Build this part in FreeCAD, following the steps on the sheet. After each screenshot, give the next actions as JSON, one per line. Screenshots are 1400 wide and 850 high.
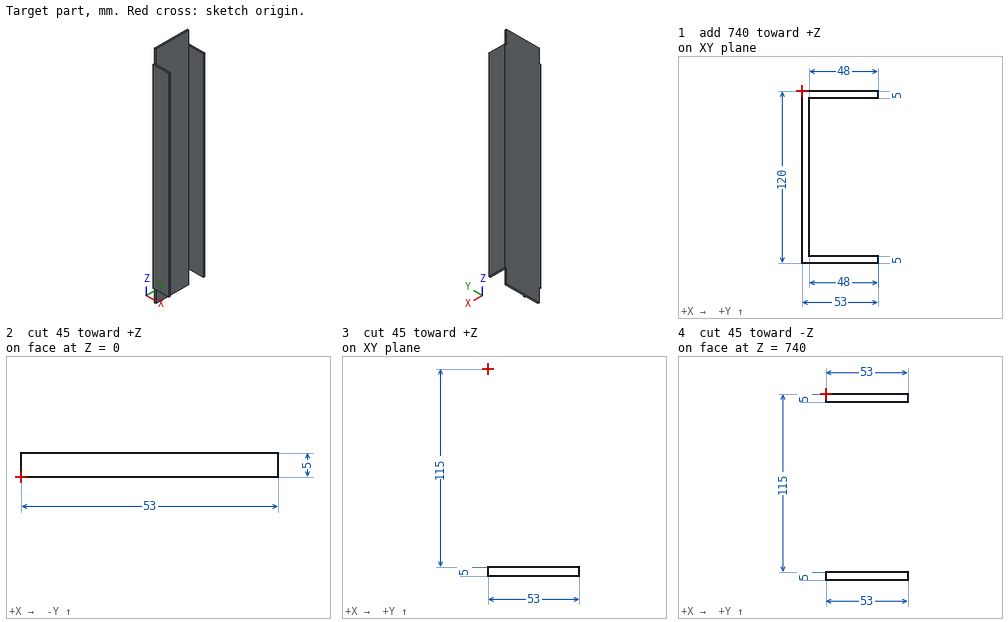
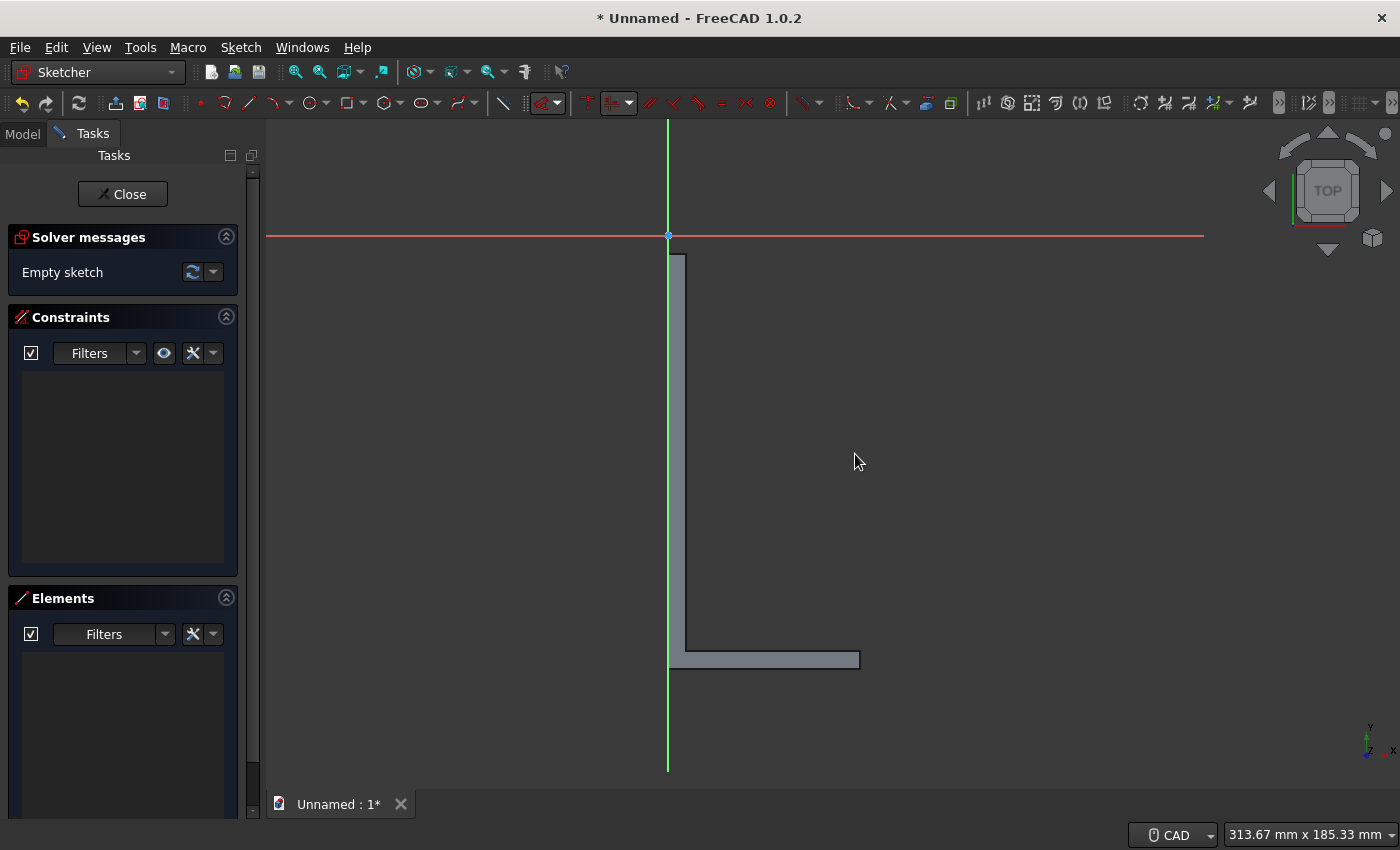
{"action": "left_click", "coordinate": [348, 104]}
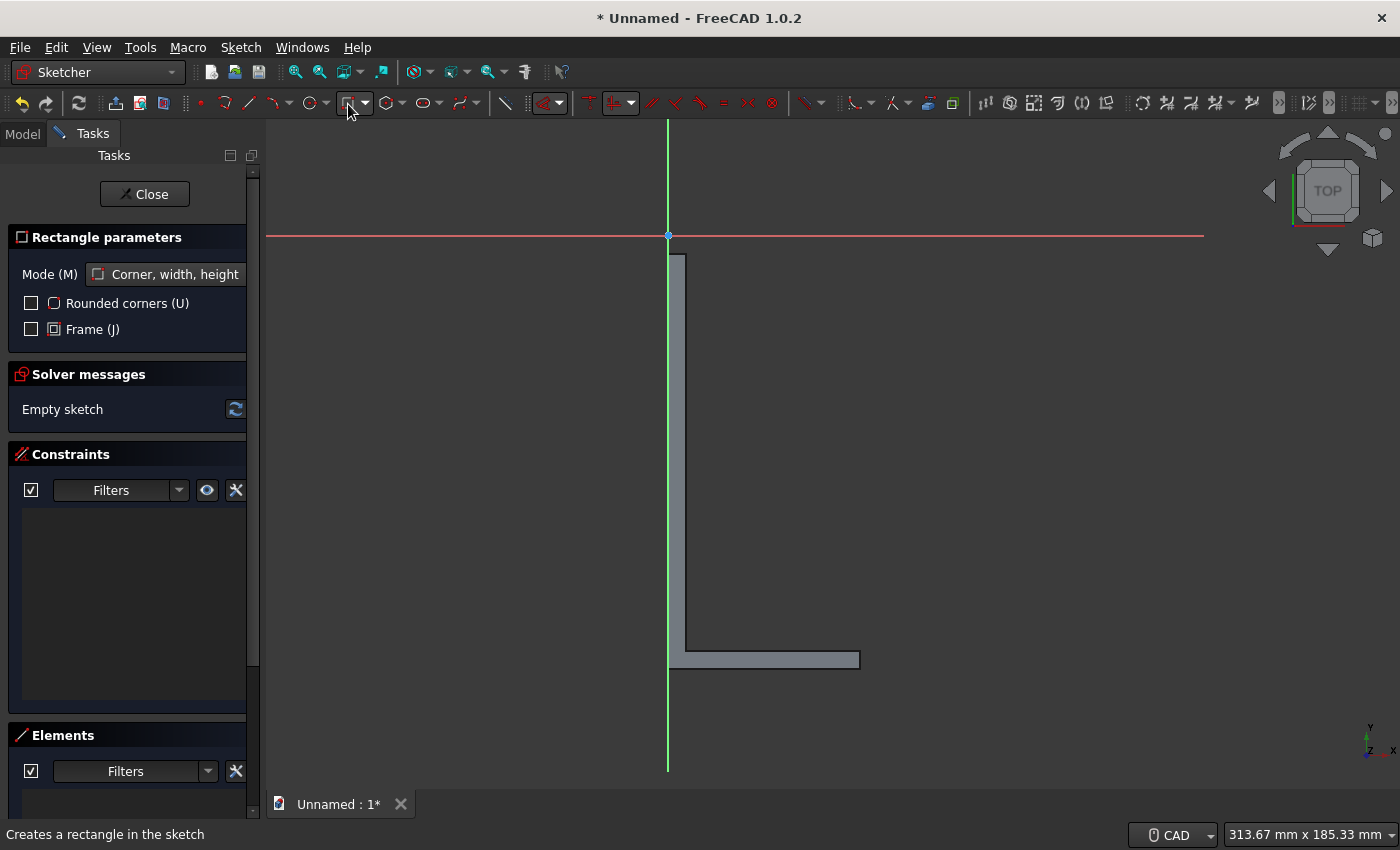
{"action": "left_click", "coordinate": [668, 651]}
{"action": "left_click", "coordinate": [860, 669]}
{"action": "key", "text": "Escape"}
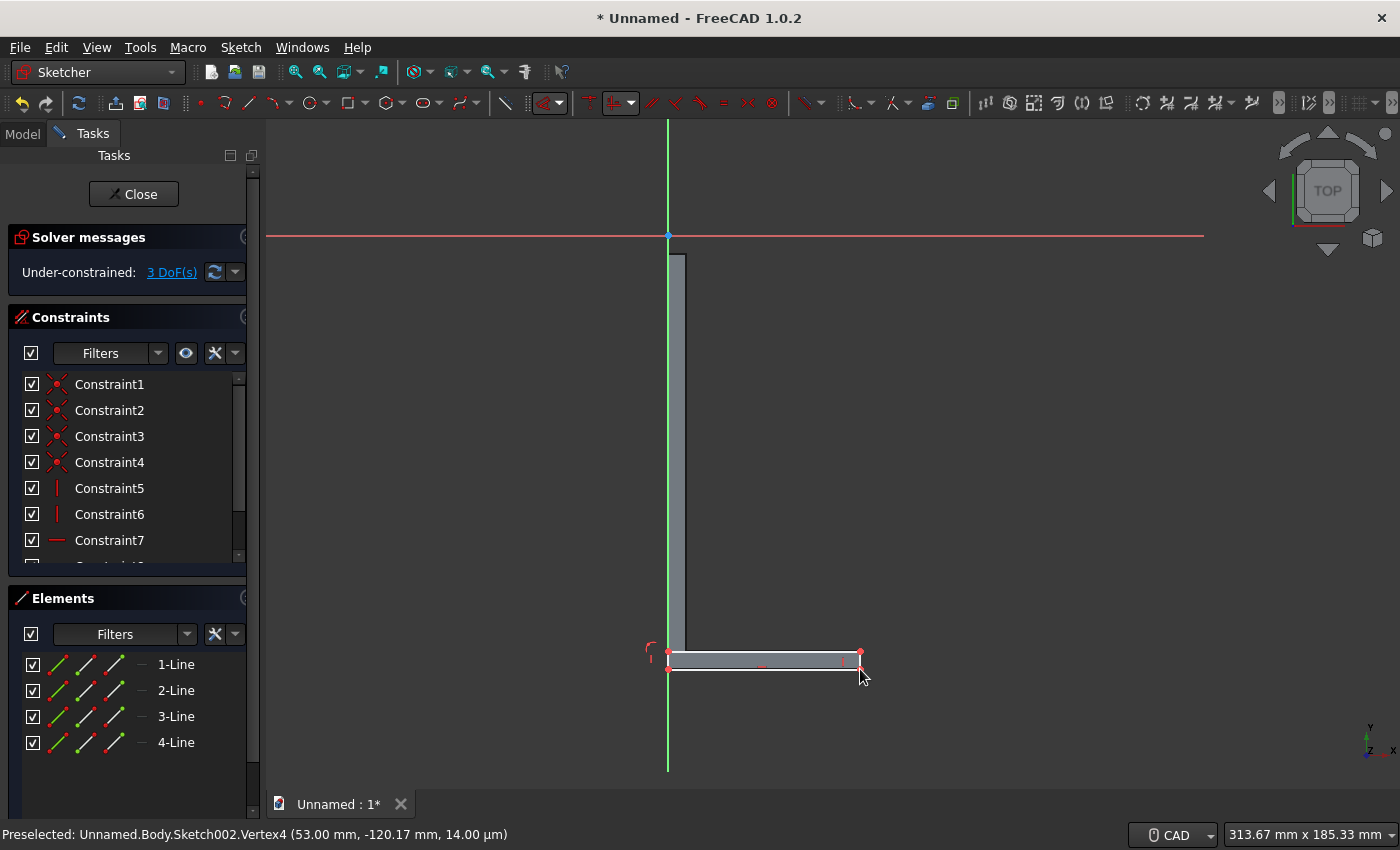
{"action": "scroll", "coordinate": [668, 661], "scroll_direction": "up", "scroll_amount": 4}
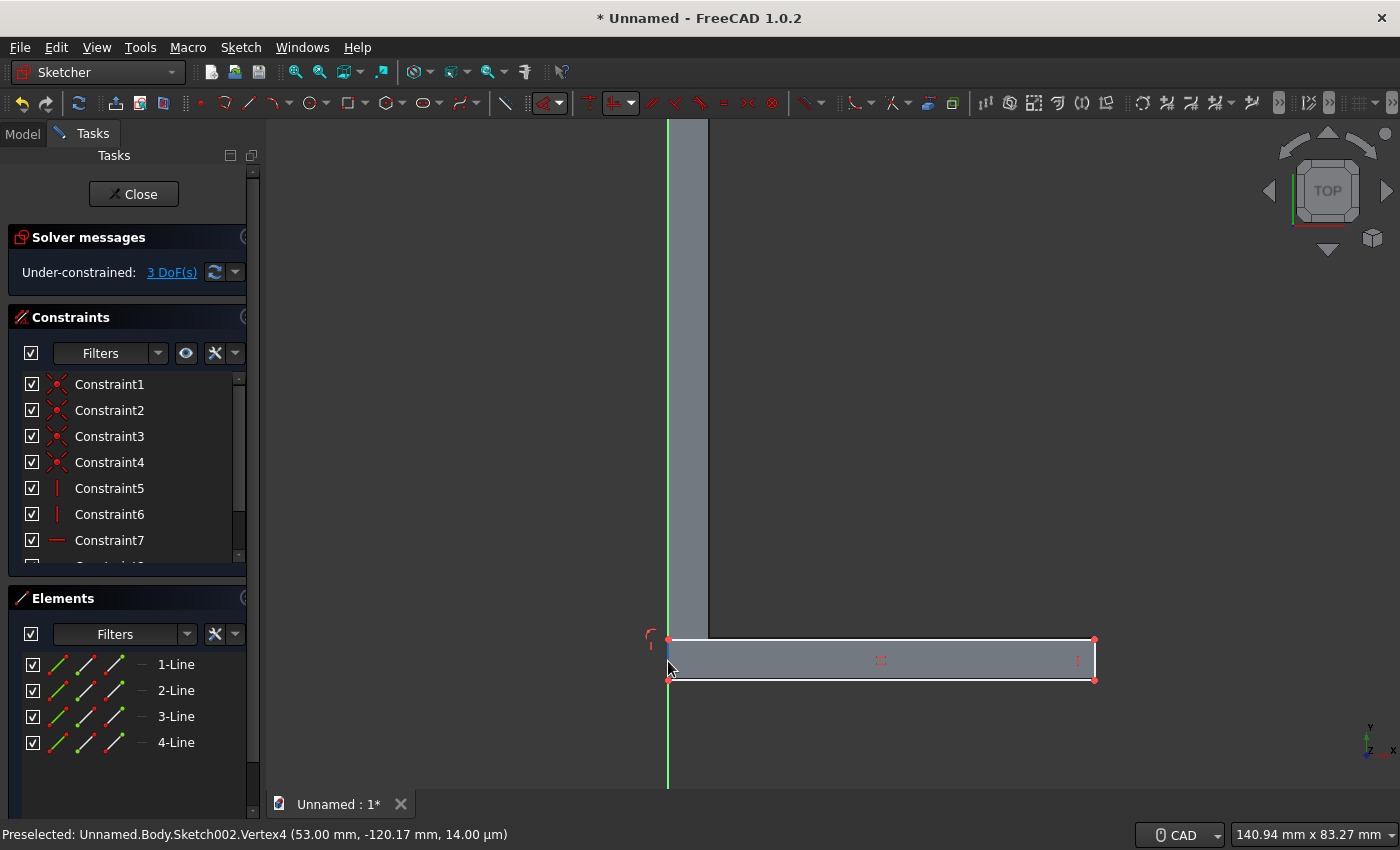
{"action": "left_click", "coordinate": [668, 660]}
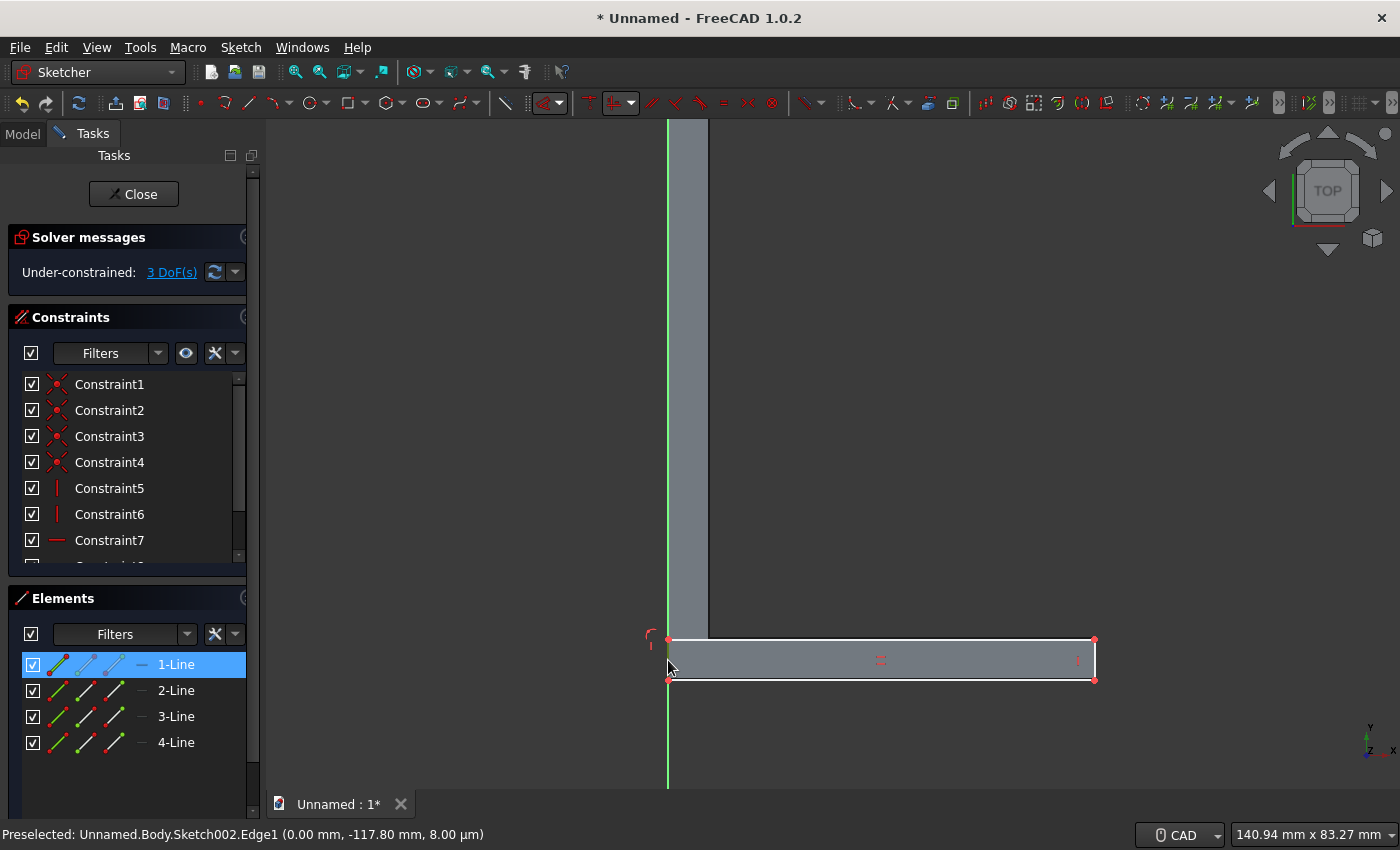
{"action": "left_click", "coordinate": [562, 104]}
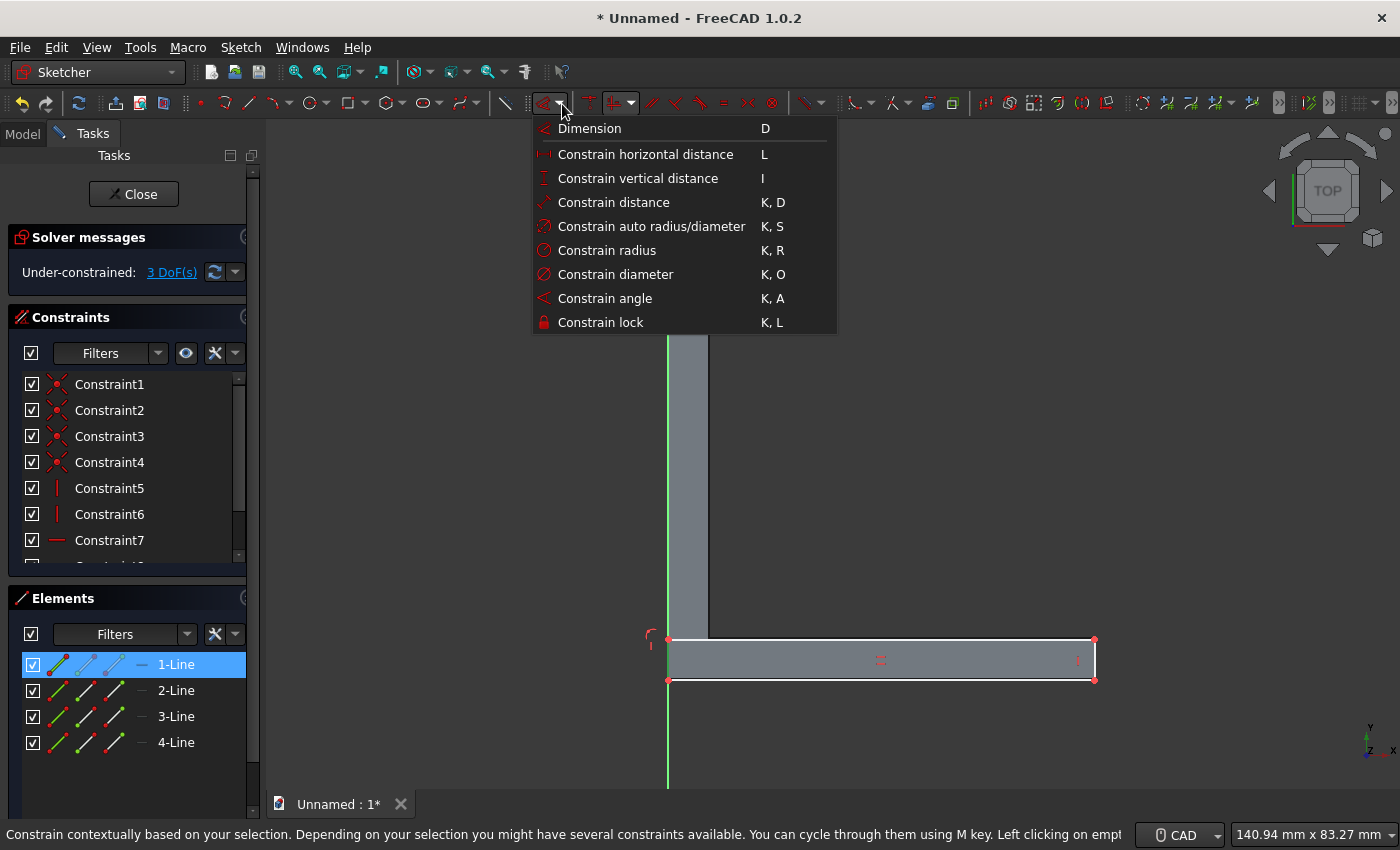
{"action": "left_click", "coordinate": [685, 178]}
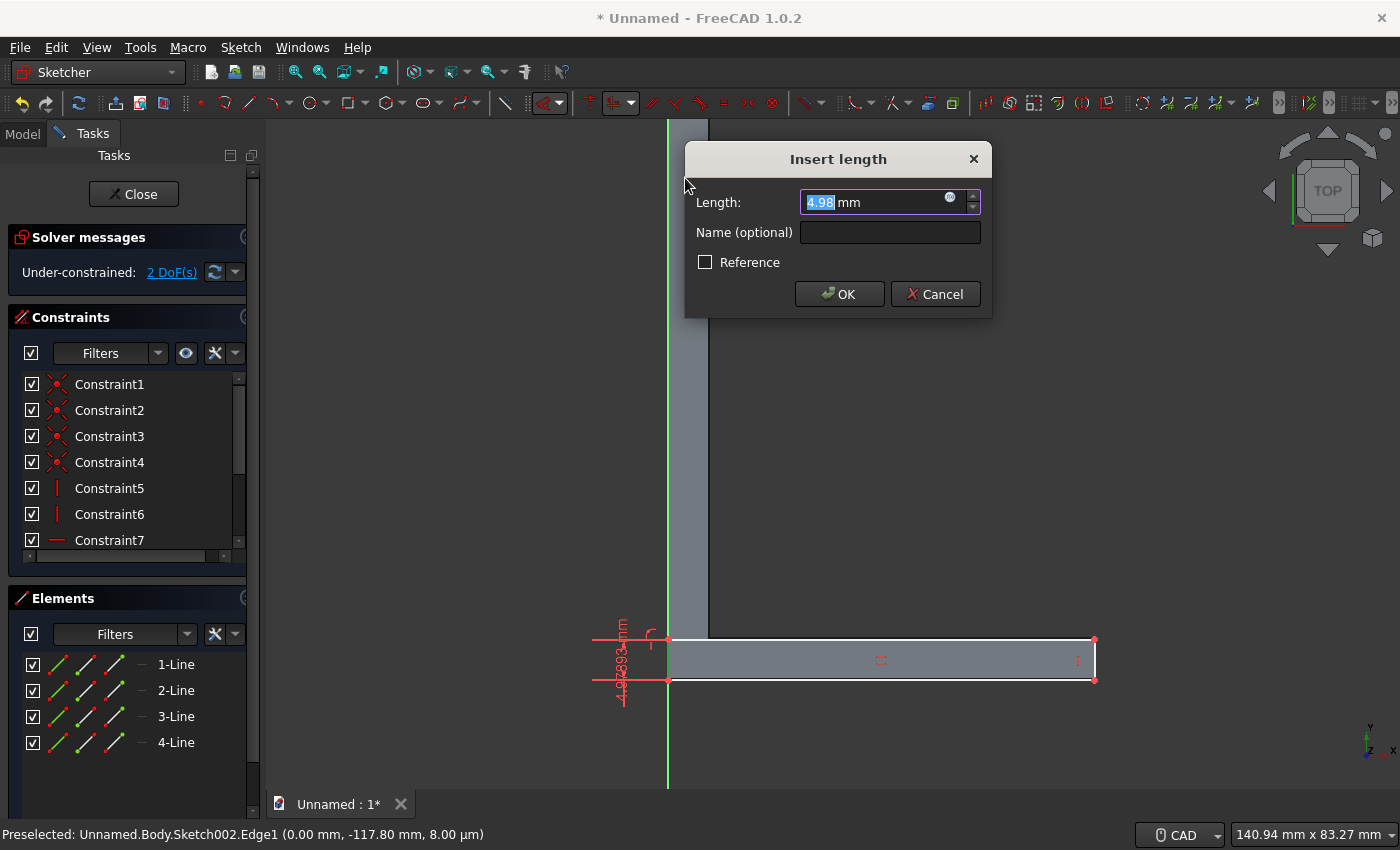
{"action": "type", "text": "5"}
{"action": "key", "text": "Return"}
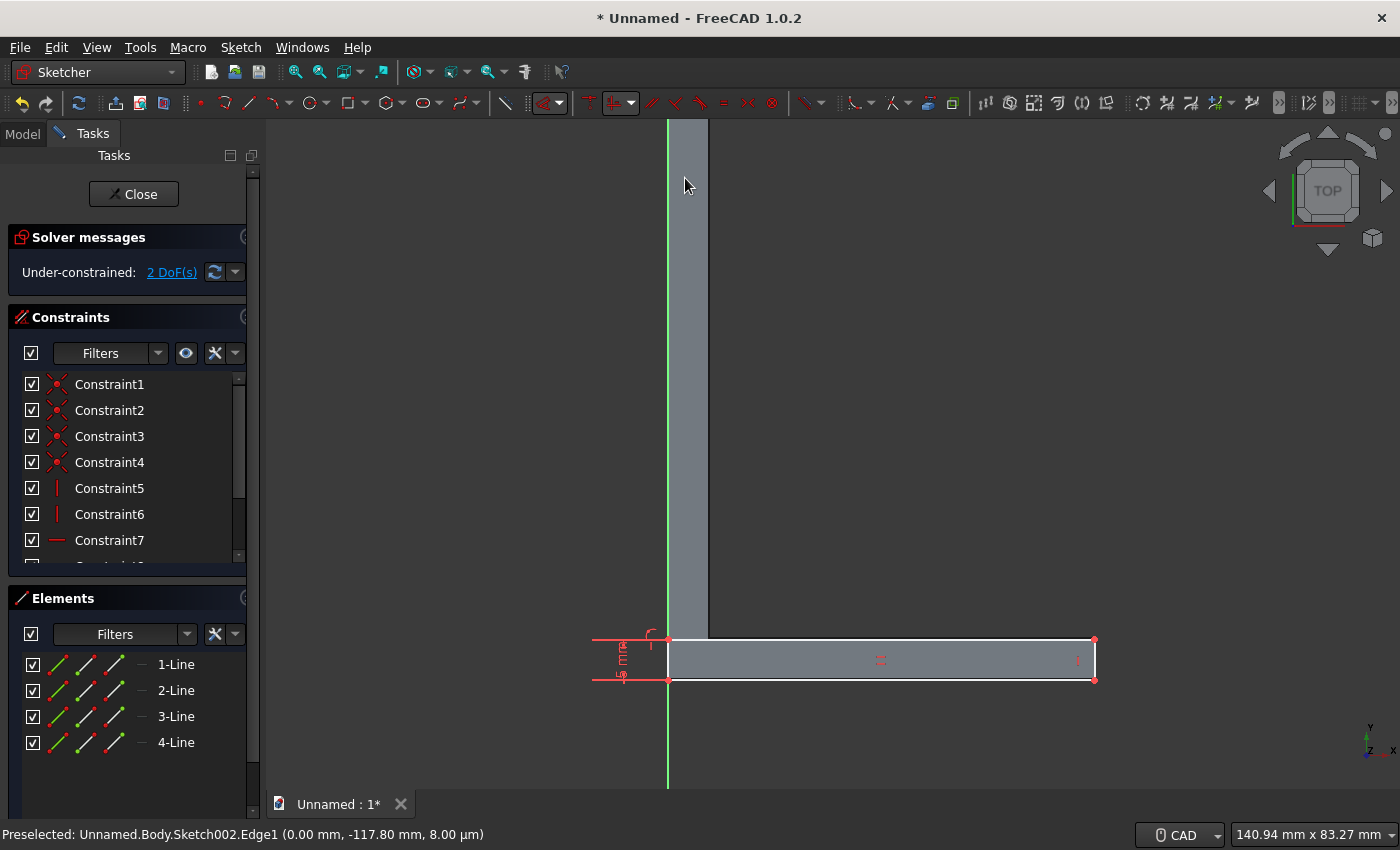
{"action": "left_click", "coordinate": [796, 680]}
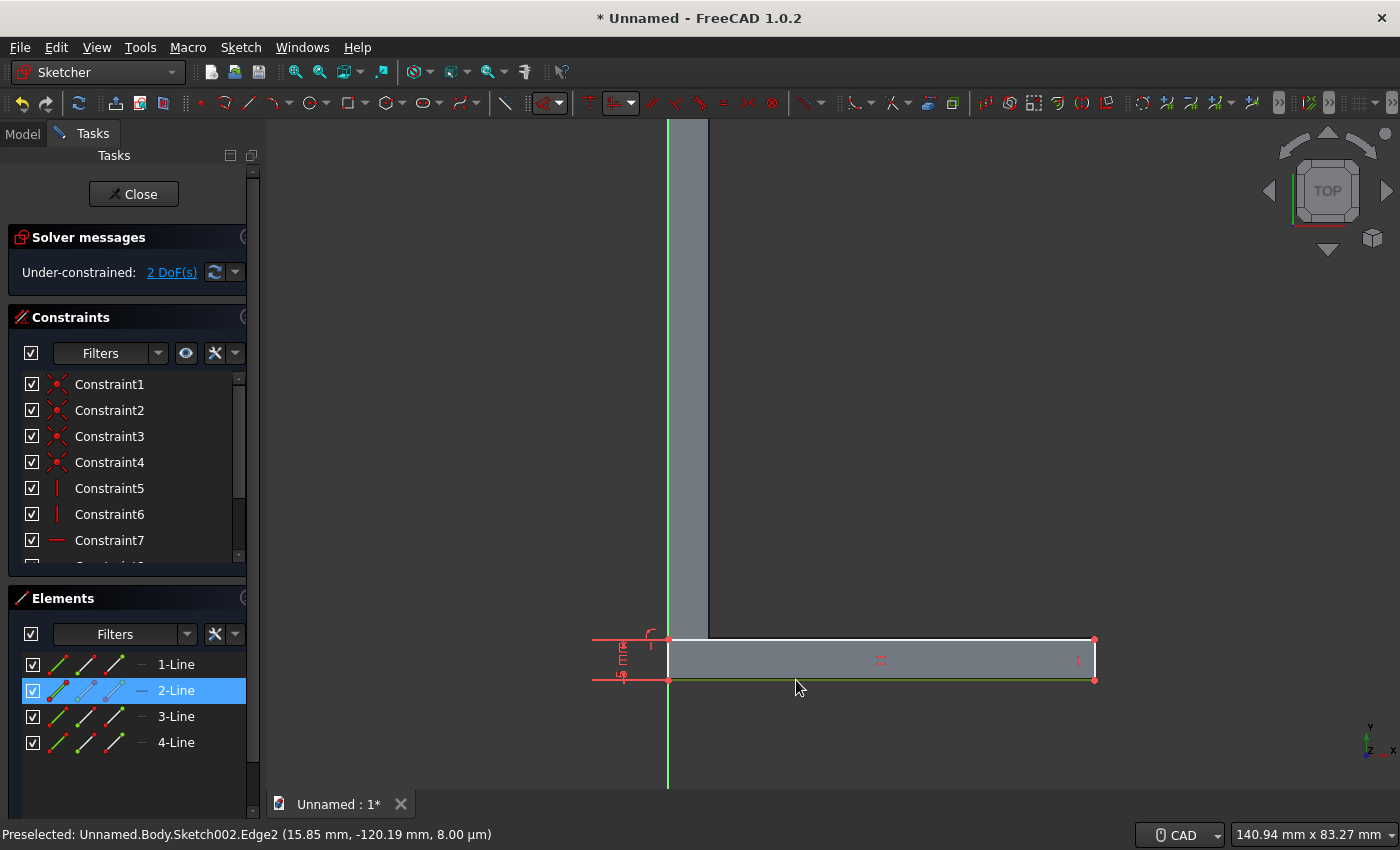
{"action": "left_click", "coordinate": [562, 104]}